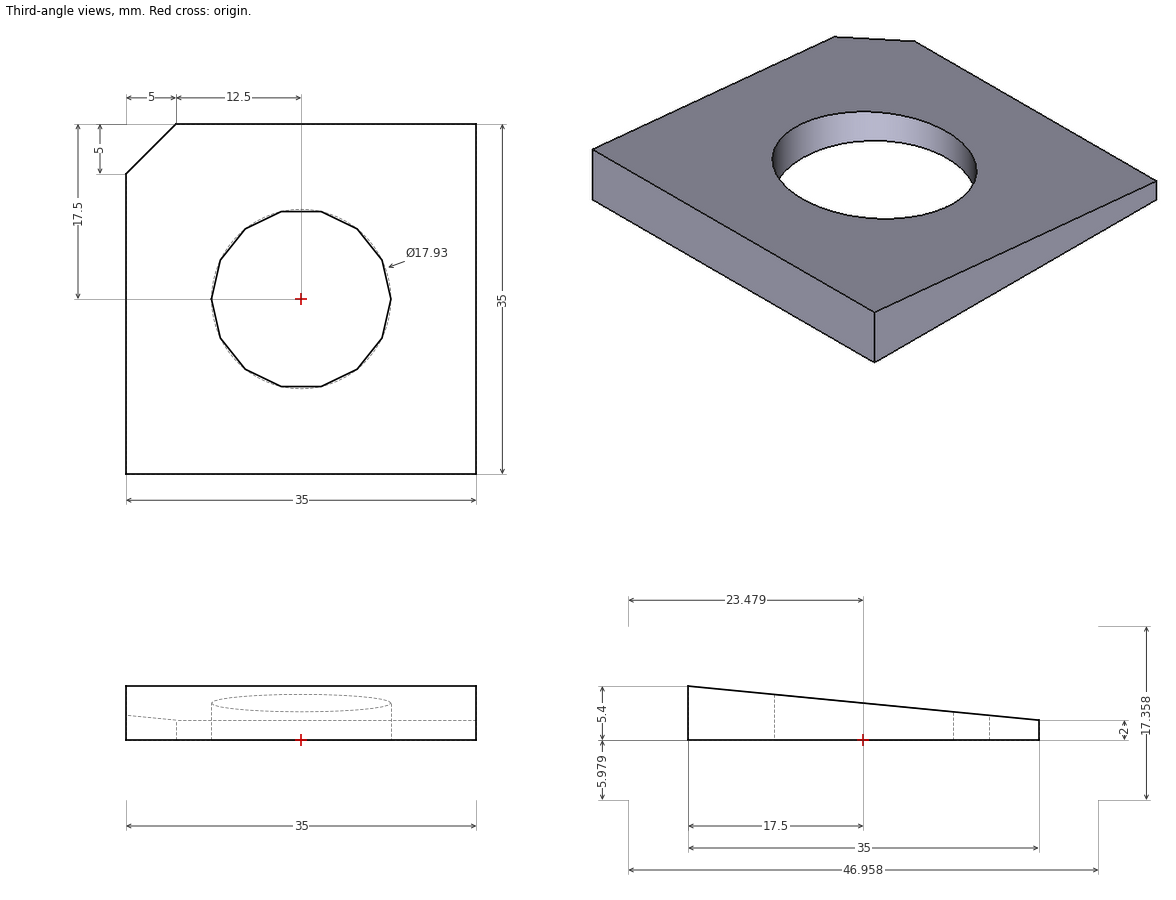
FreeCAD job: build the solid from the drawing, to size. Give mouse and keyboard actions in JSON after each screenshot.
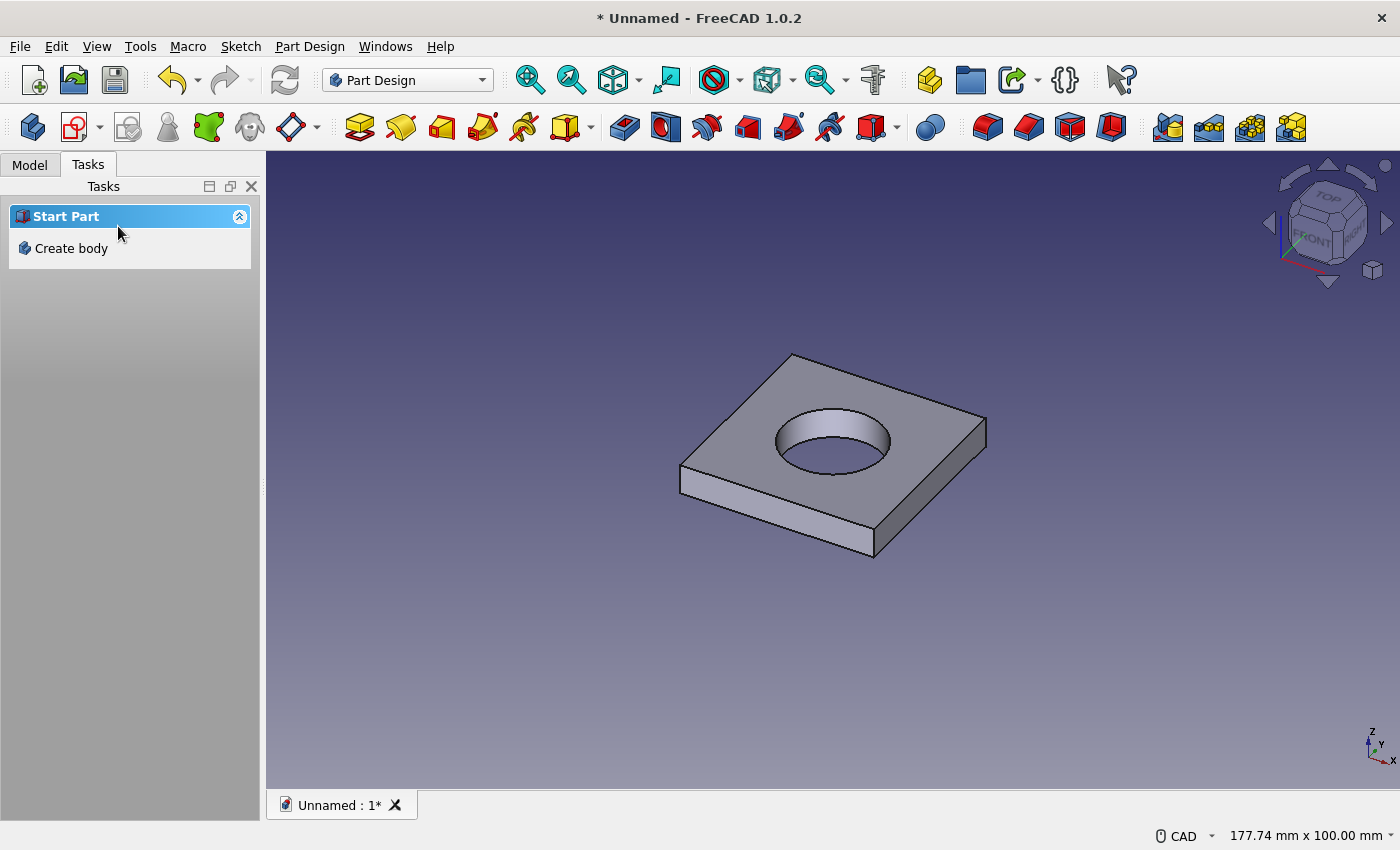
{"action": "key", "text": "v f"}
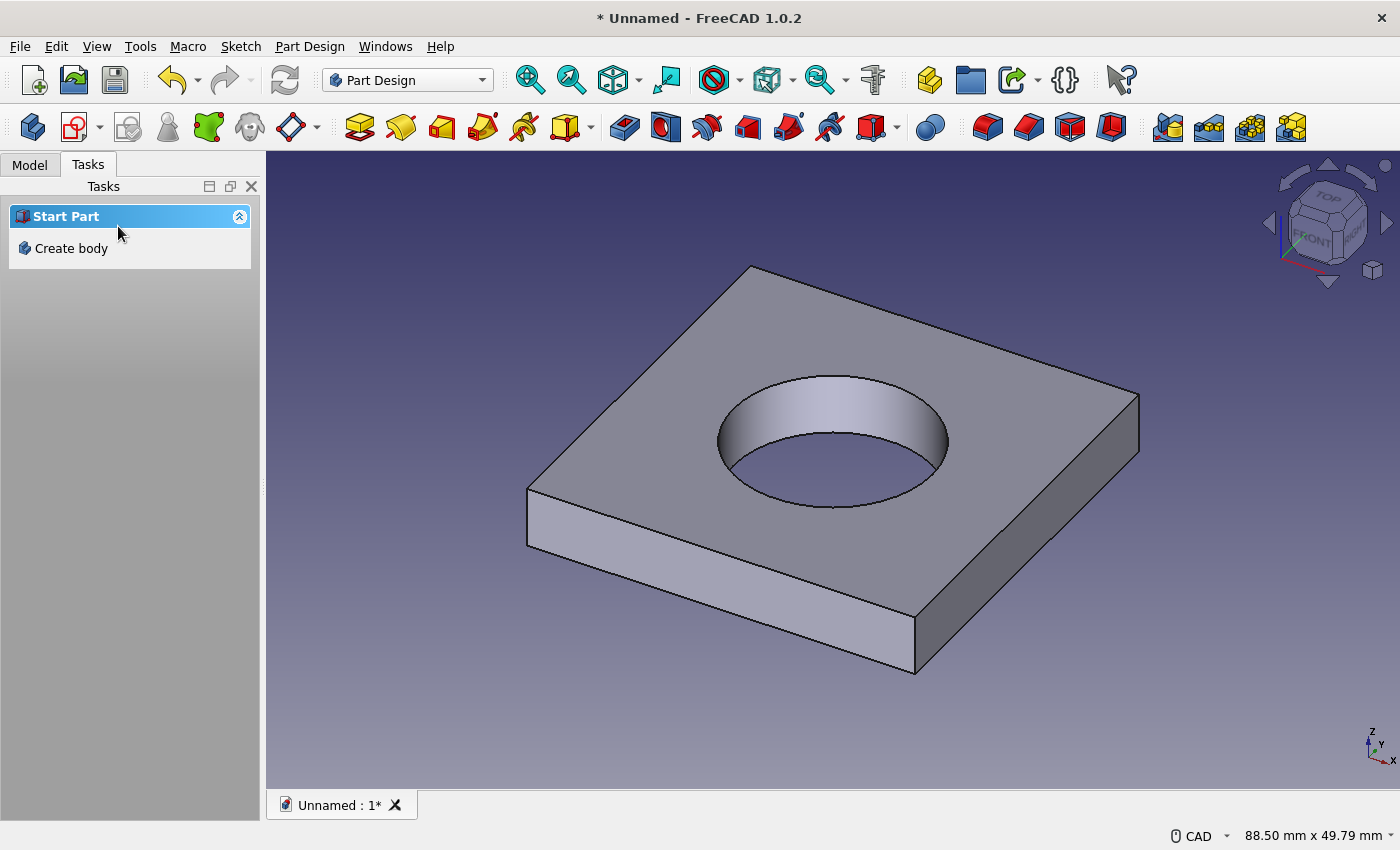
{"action": "left_click", "coordinate": [1091, 470]}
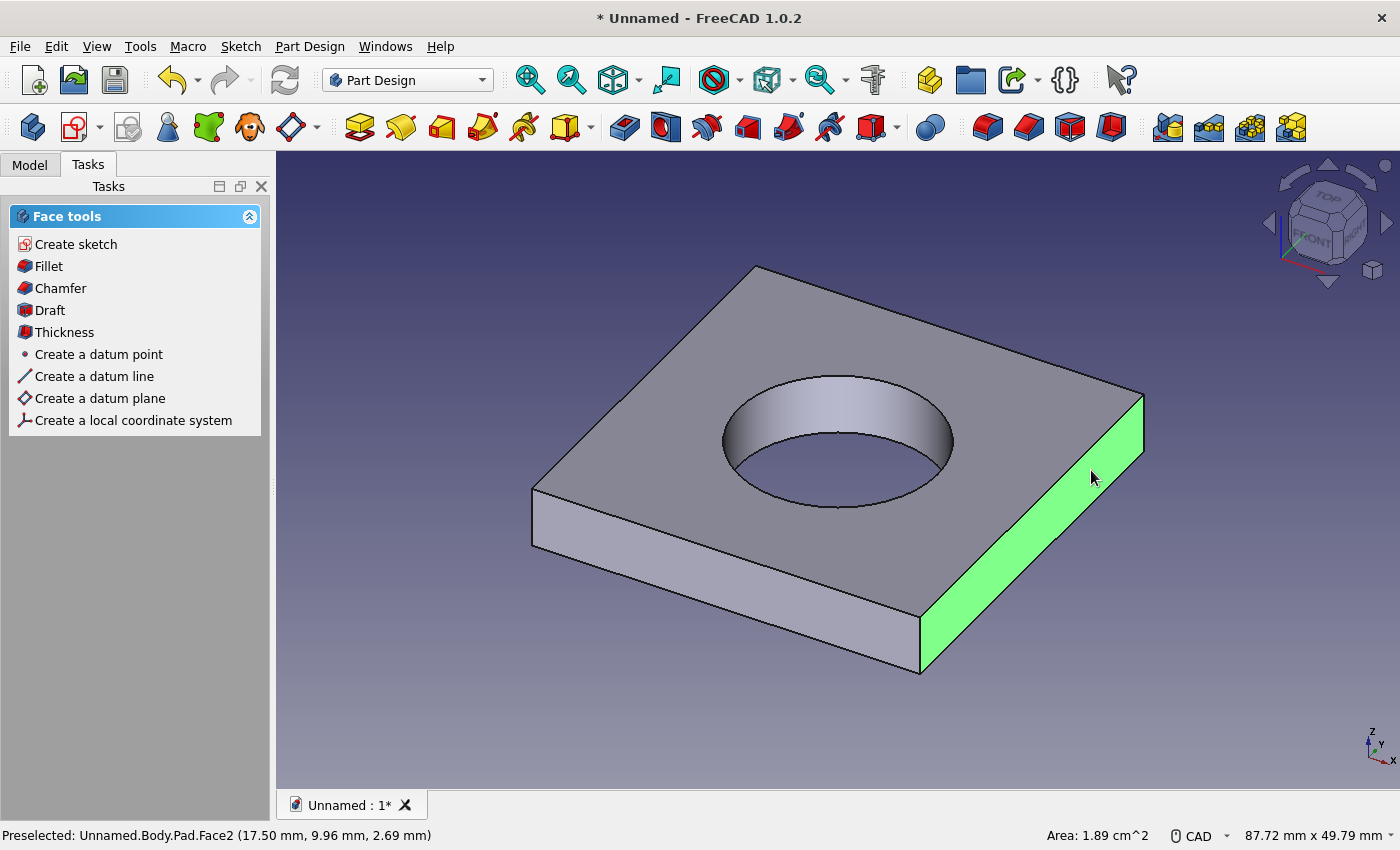
{"action": "left_click", "coordinate": [74, 128]}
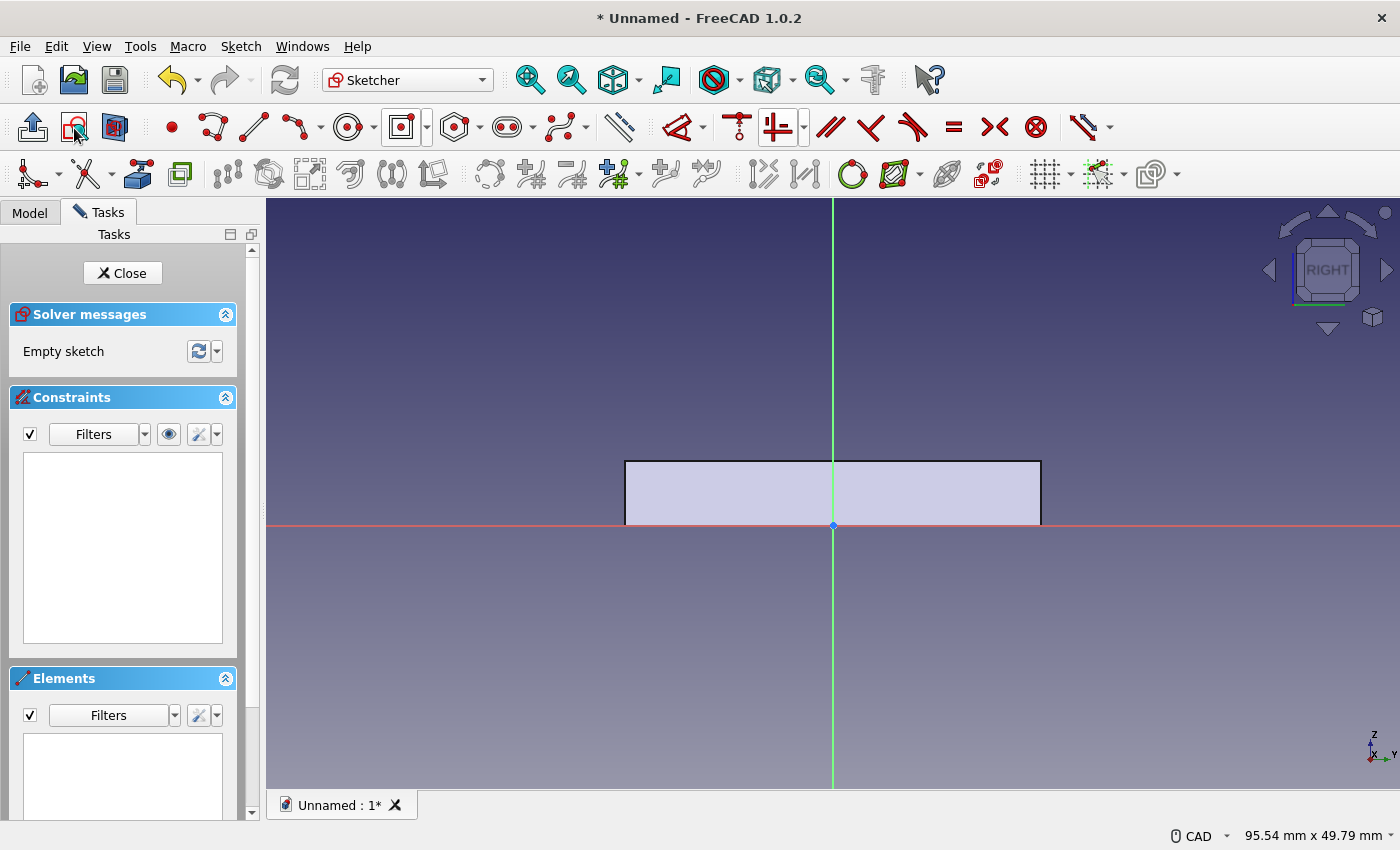
{"action": "key", "text": "g r"}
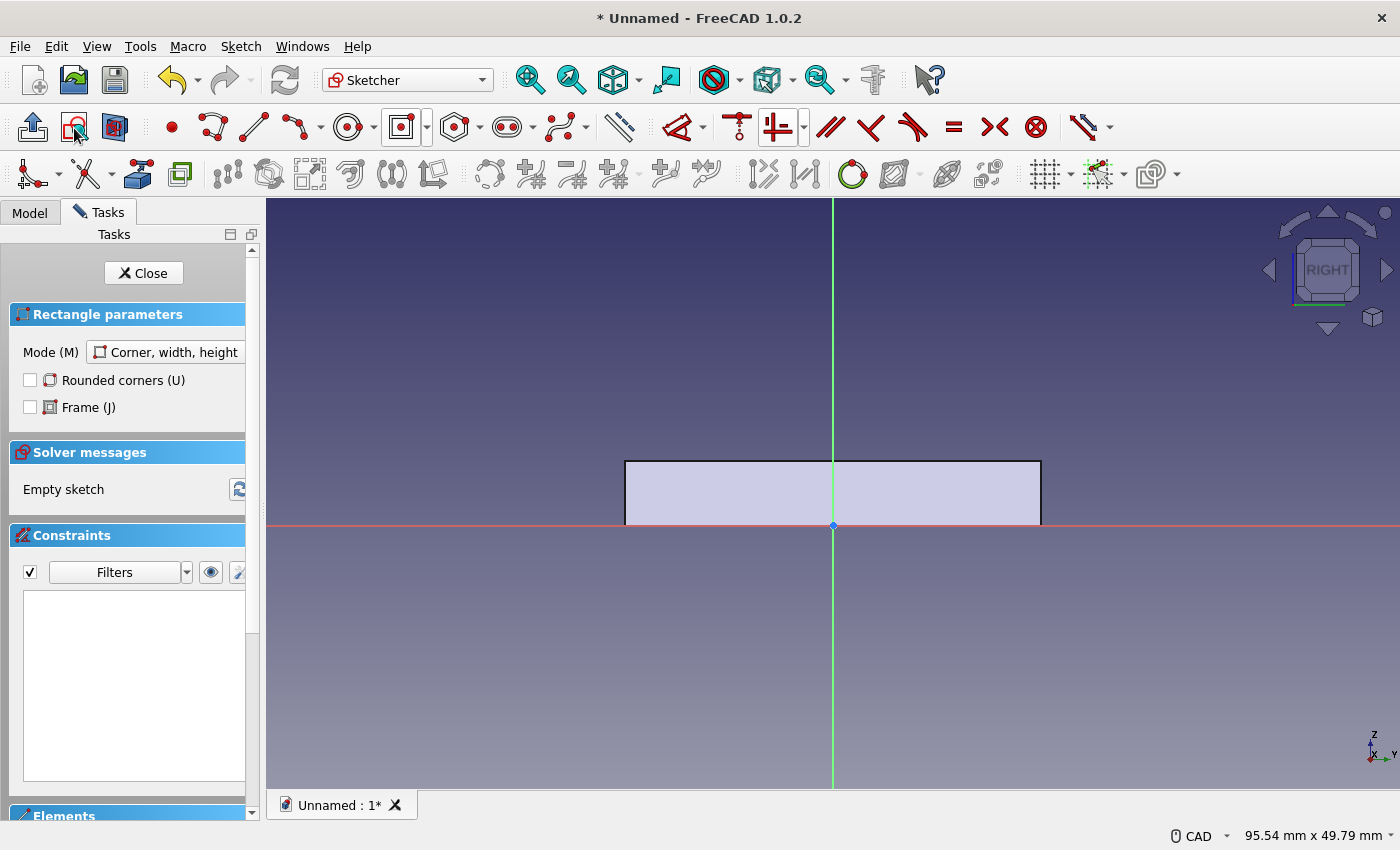
{"action": "left_click", "coordinate": [554, 390]}
{"action": "mouse_move", "coordinate": [1112, 597]}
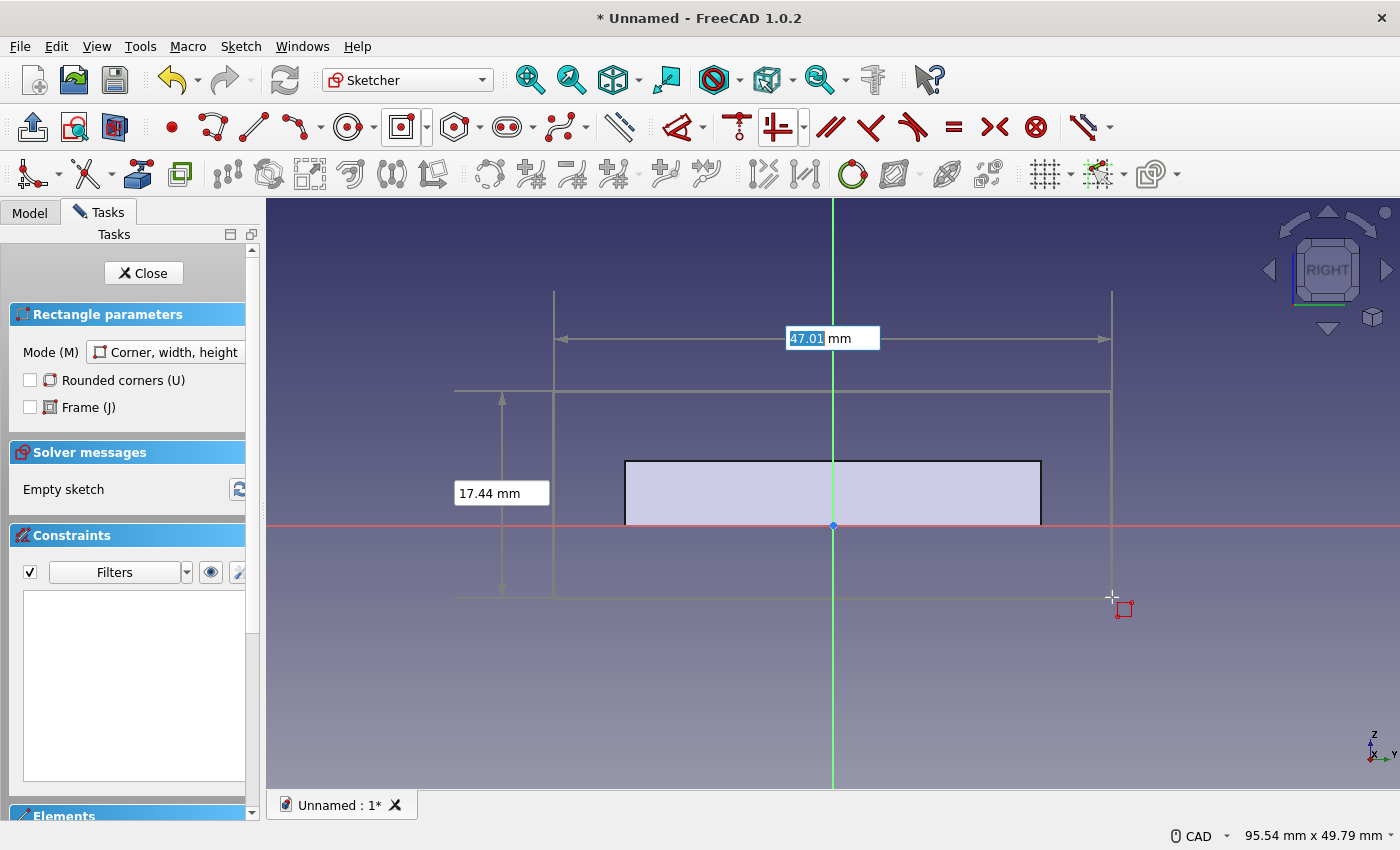
{"action": "type", "text": "46.958"}
{"action": "key", "text": "Tab"}
{"action": "type", "text": "17.358"}
{"action": "key", "text": "Return"}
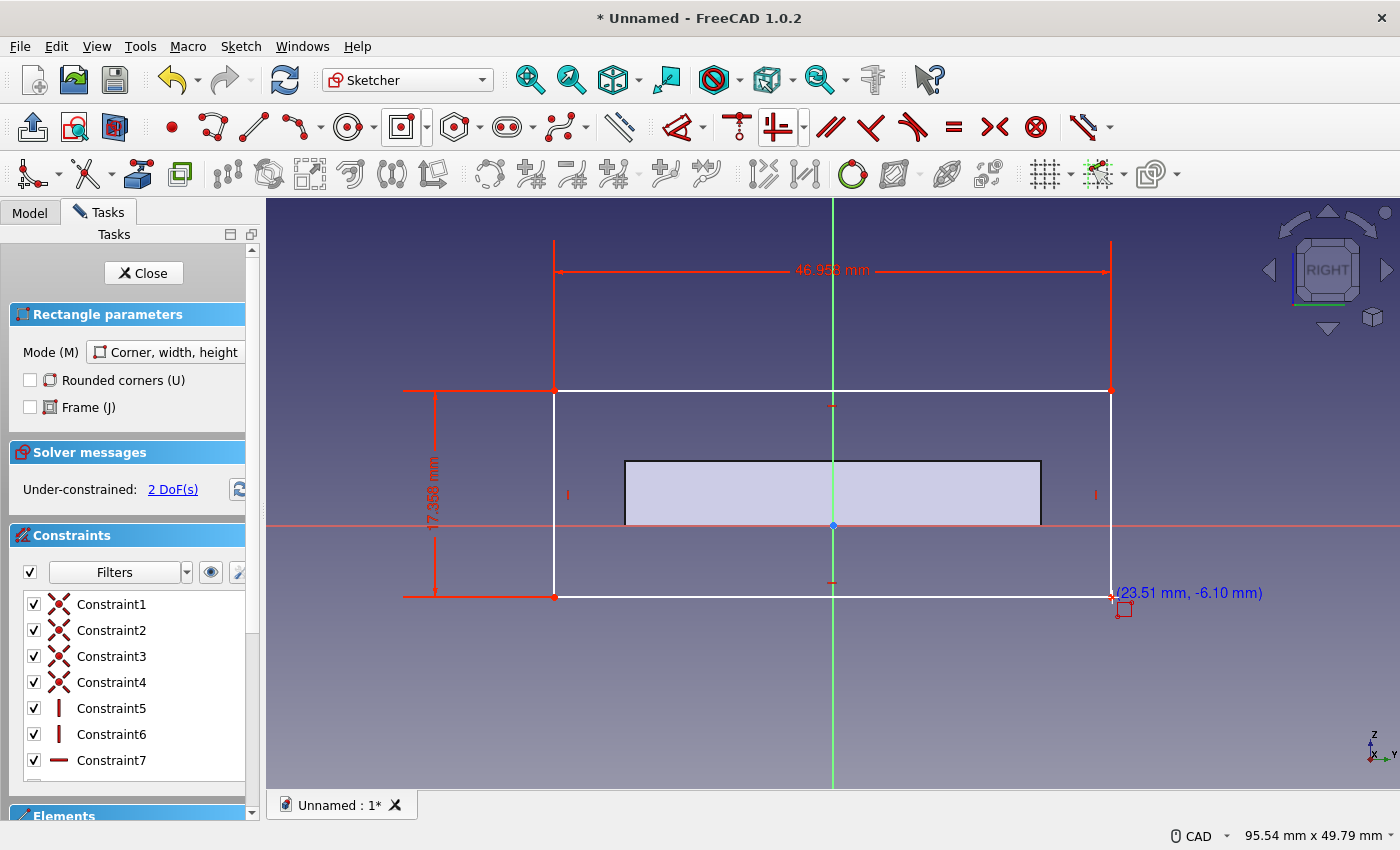
{"action": "key", "text": "g m"}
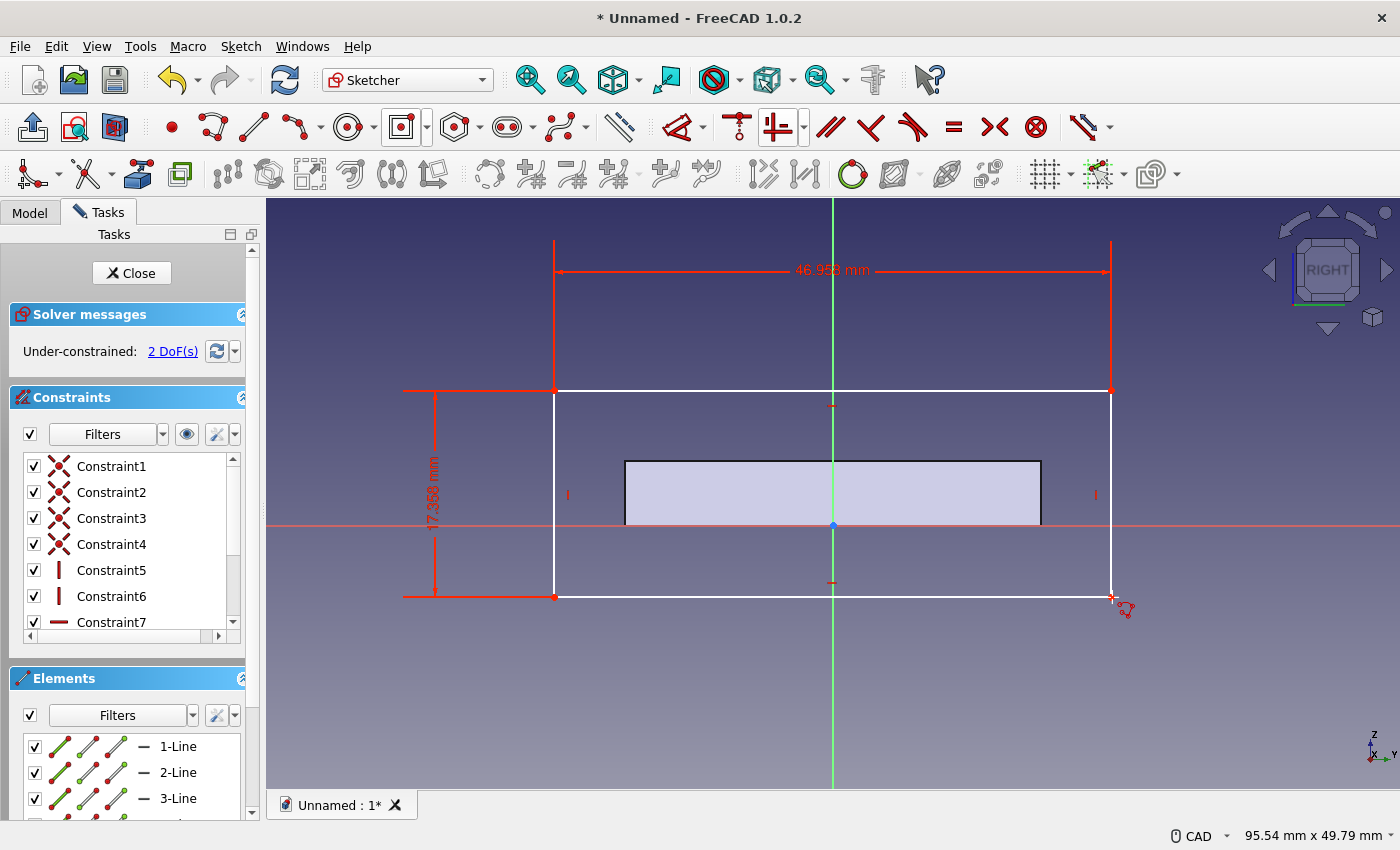
{"action": "left_click", "coordinate": [625, 526]}
{"action": "left_click", "coordinate": [625, 461]}
{"action": "left_click", "coordinate": [1041, 502]}
{"action": "left_click", "coordinate": [1041, 517]}
{"action": "left_click", "coordinate": [625, 526]}
{"action": "key", "text": "Escape"}
{"action": "key", "text": "Escape"}